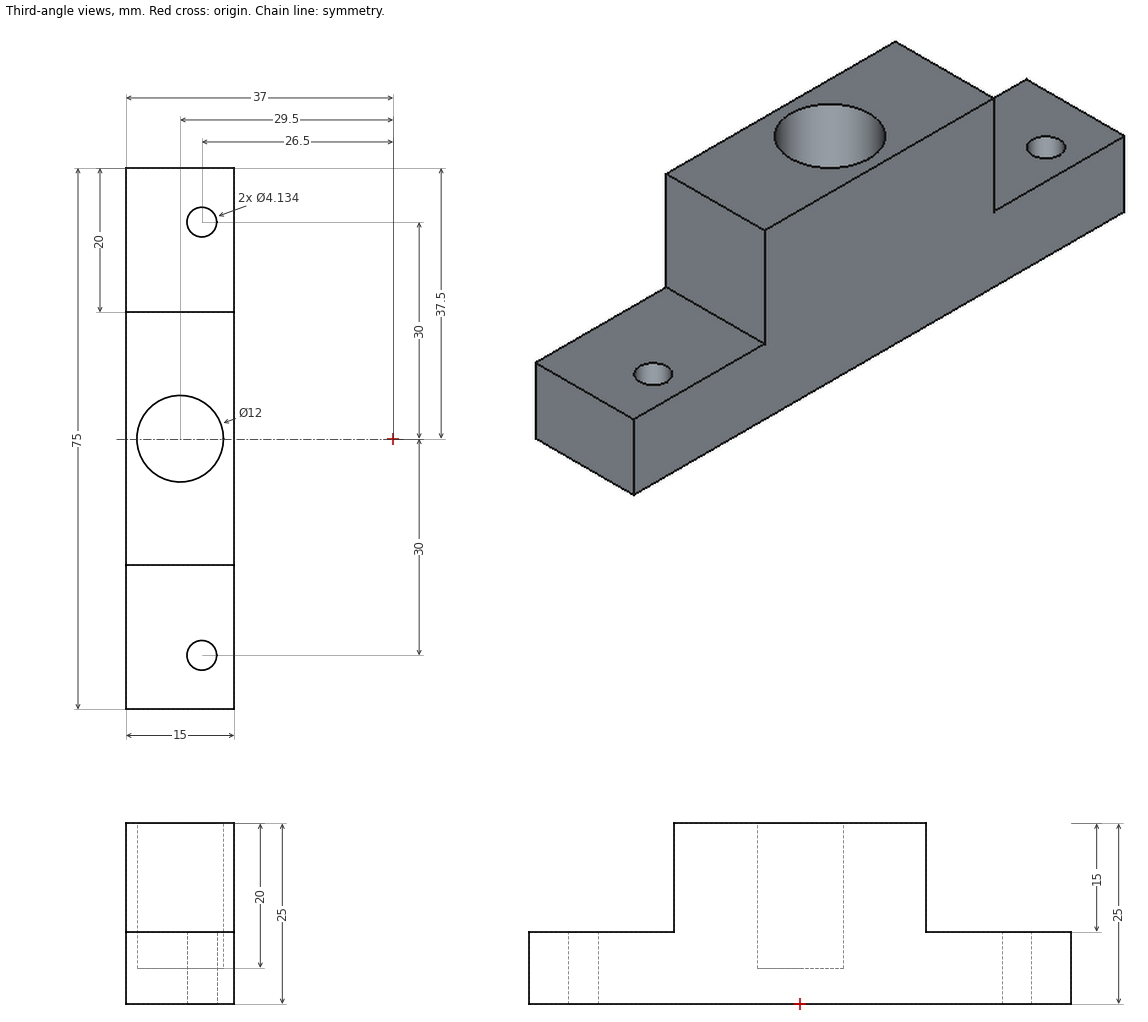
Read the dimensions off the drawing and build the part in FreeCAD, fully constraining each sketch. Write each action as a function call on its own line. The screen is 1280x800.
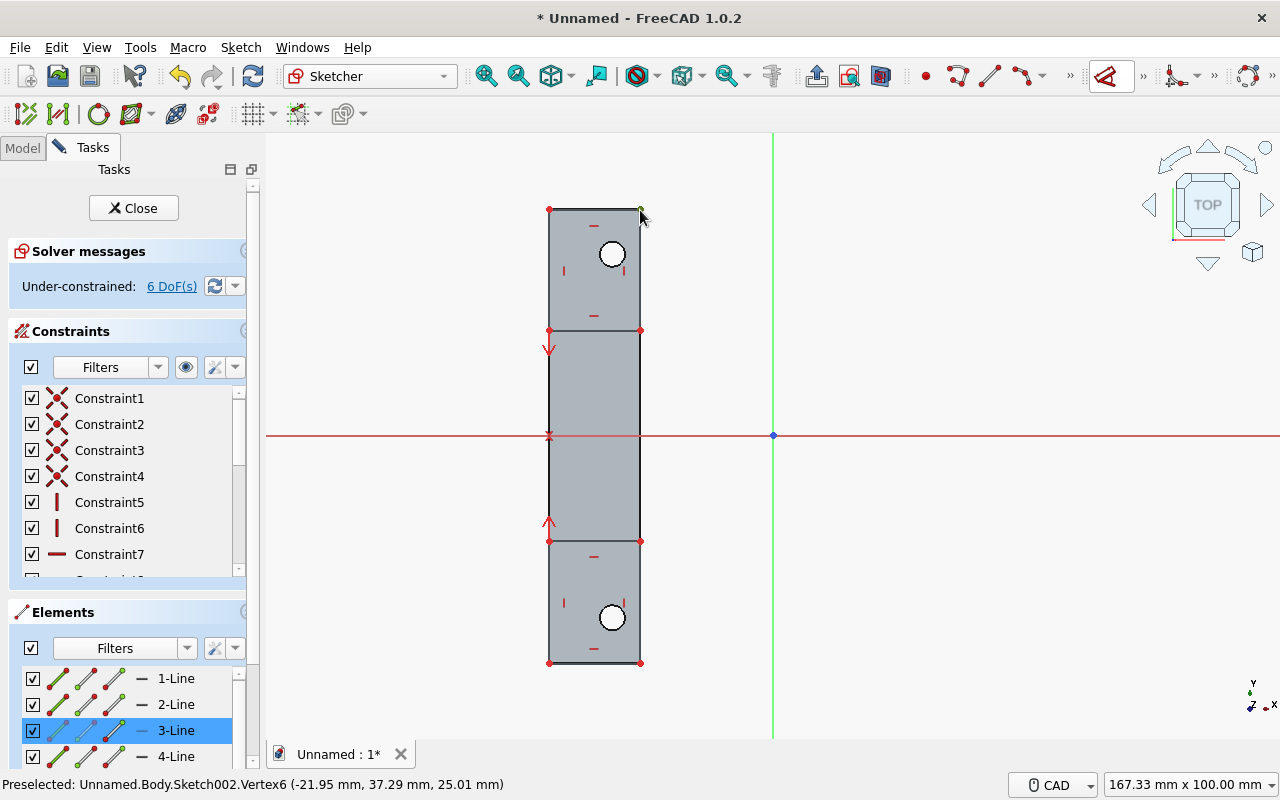
click(640, 664)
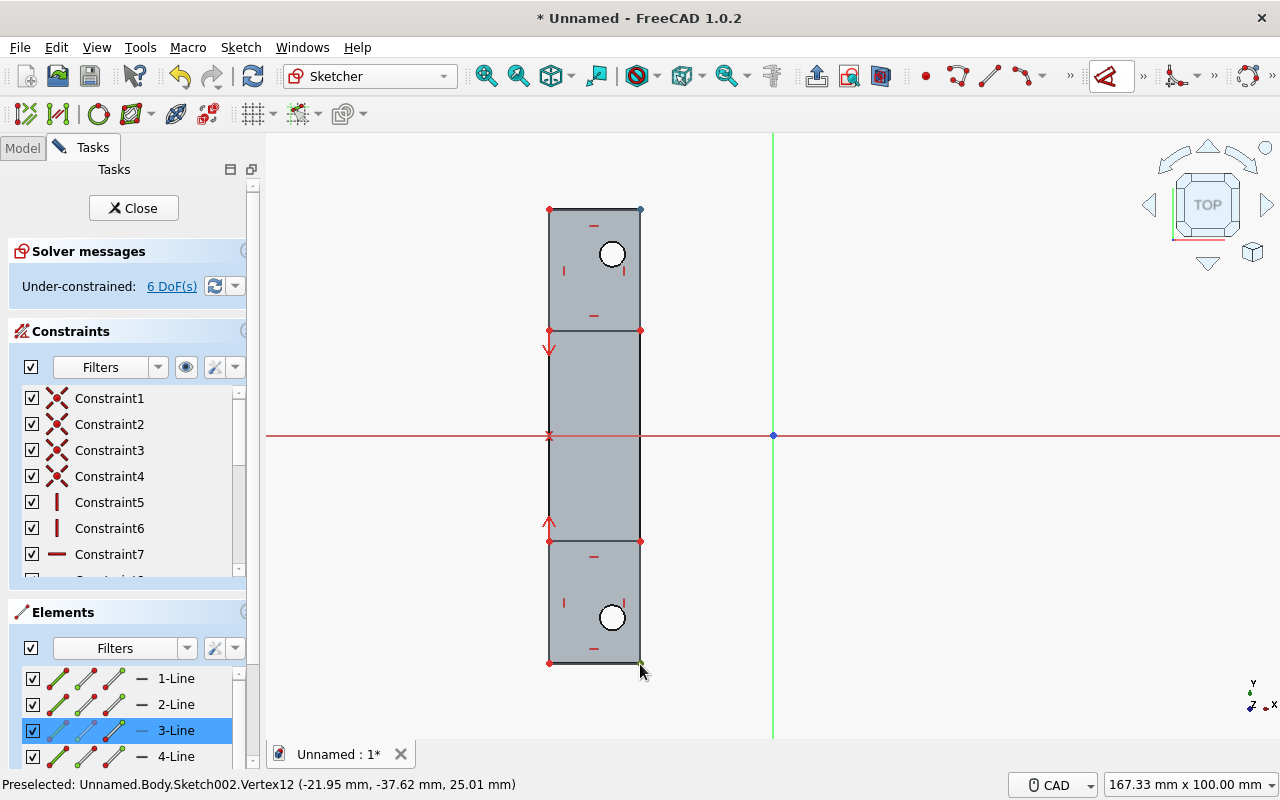
click(353, 436)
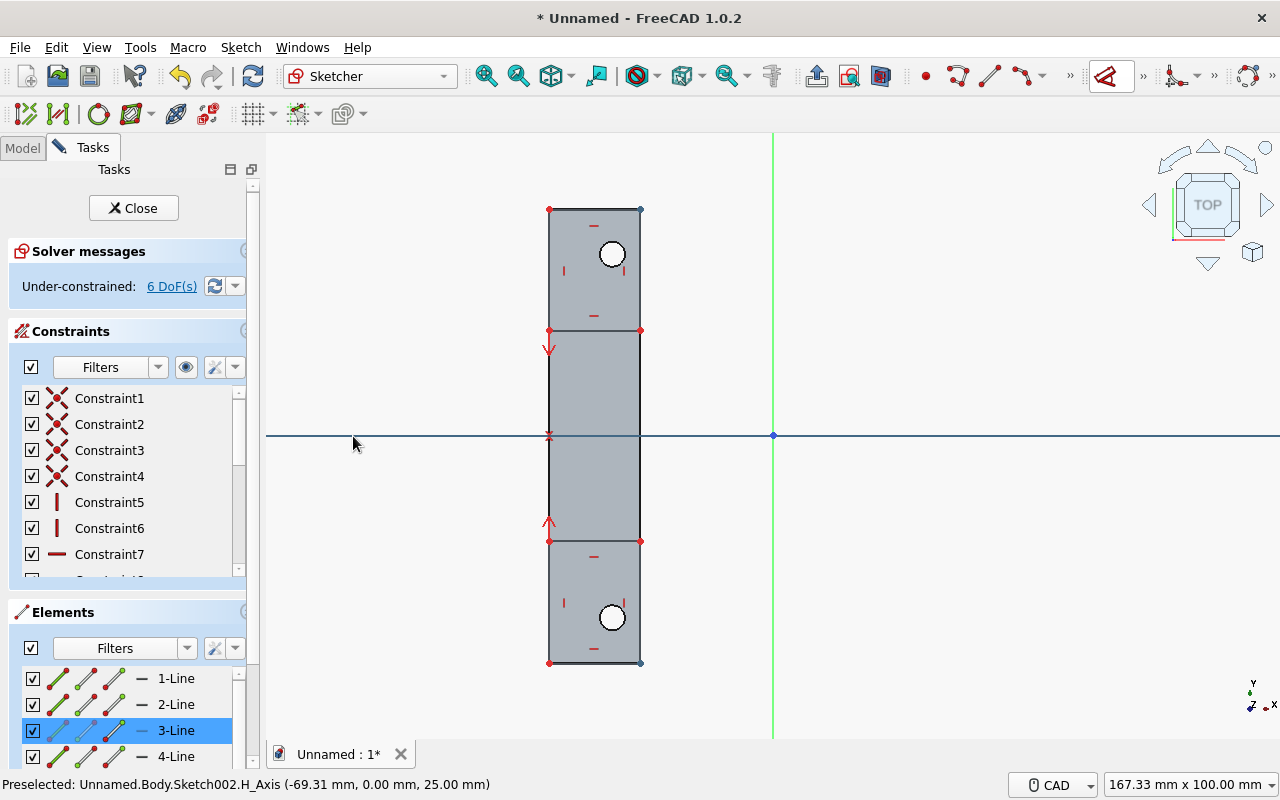
key(s)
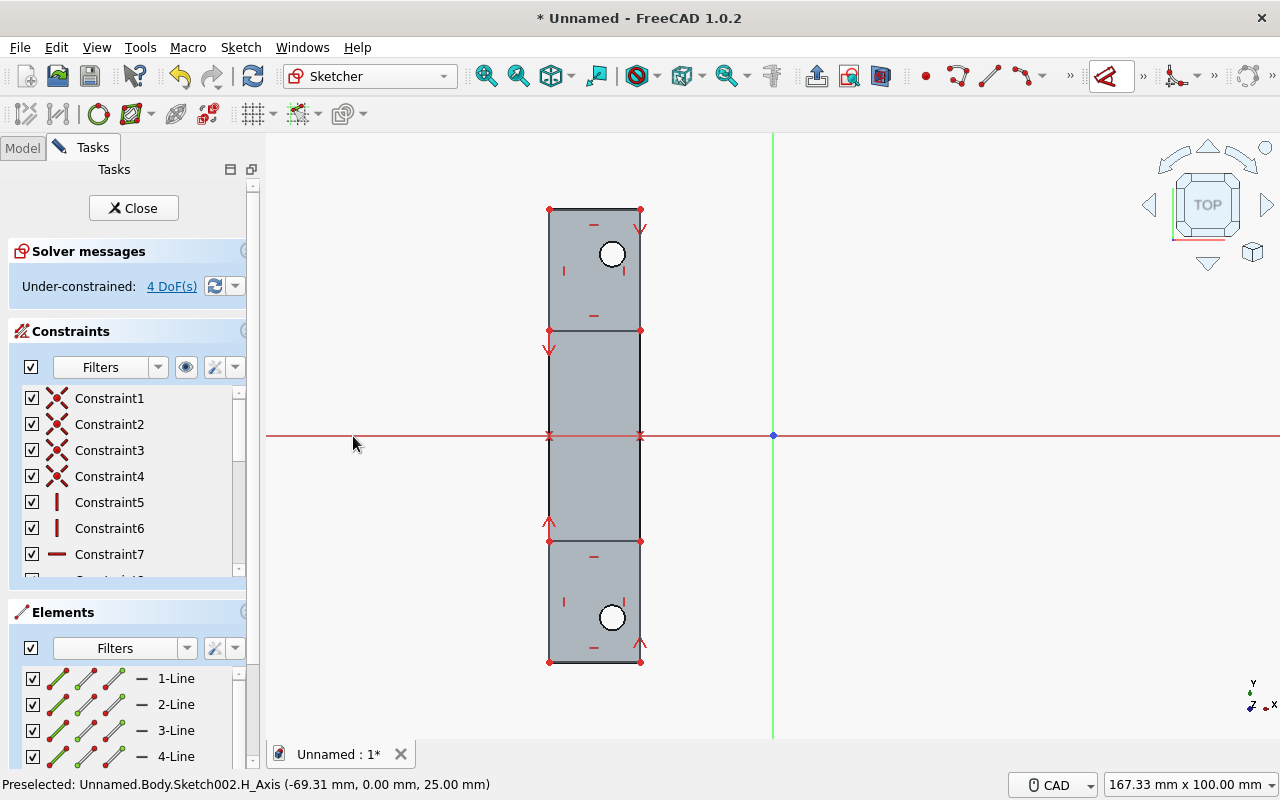
click(549, 246)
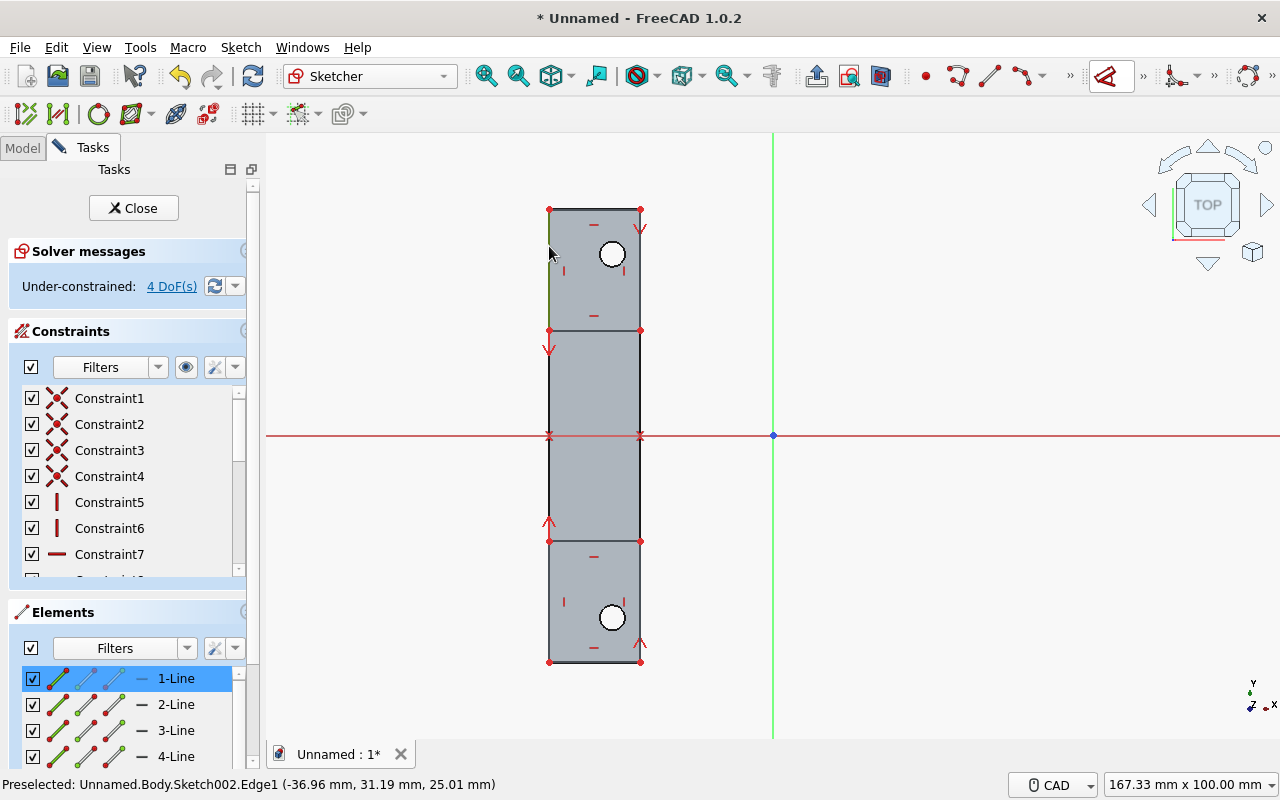
key(i)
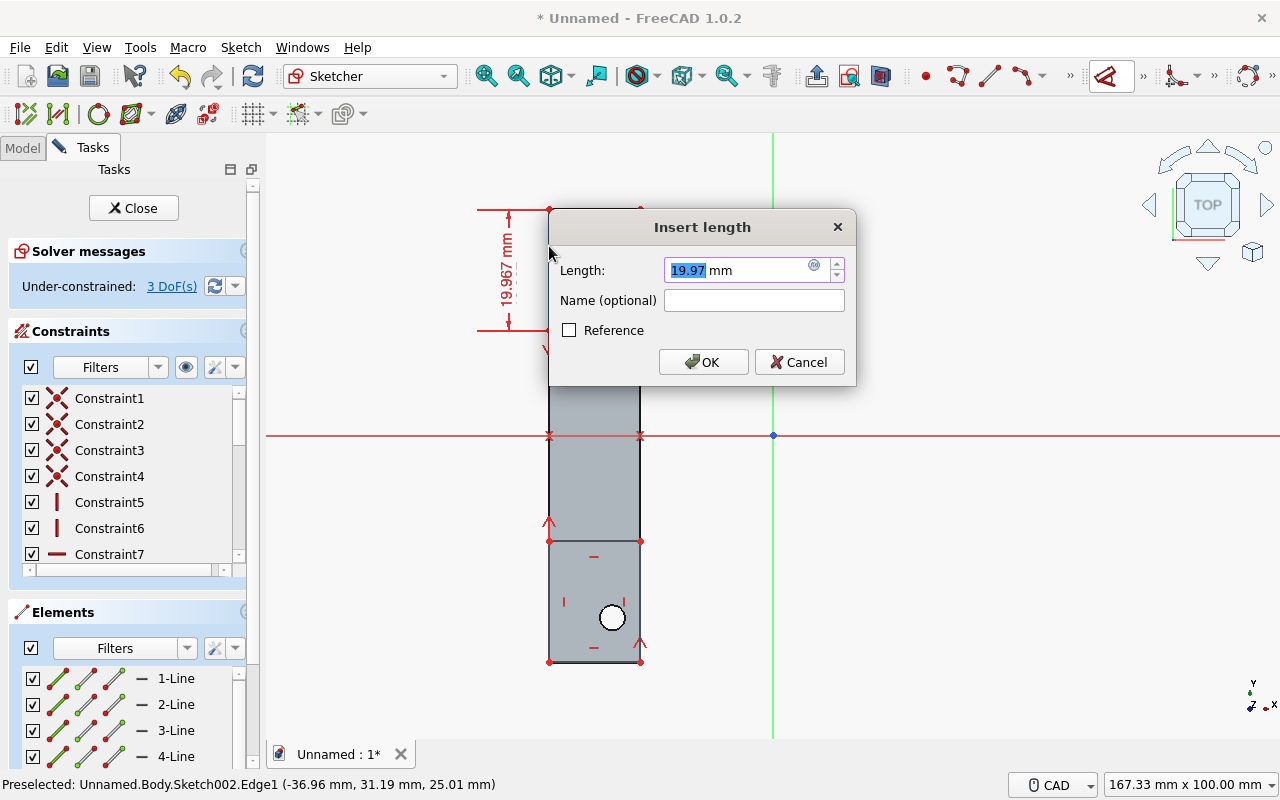
text(20)
key(Return)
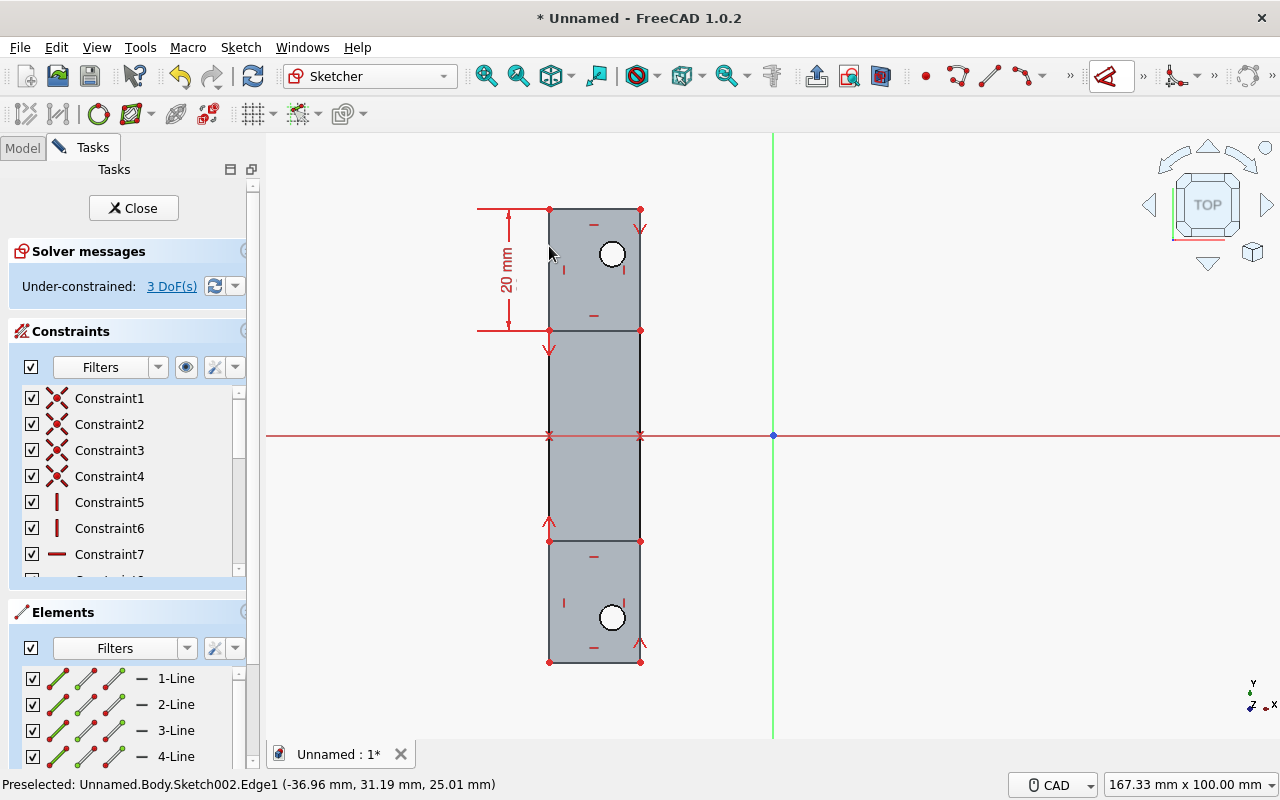
click(576, 331)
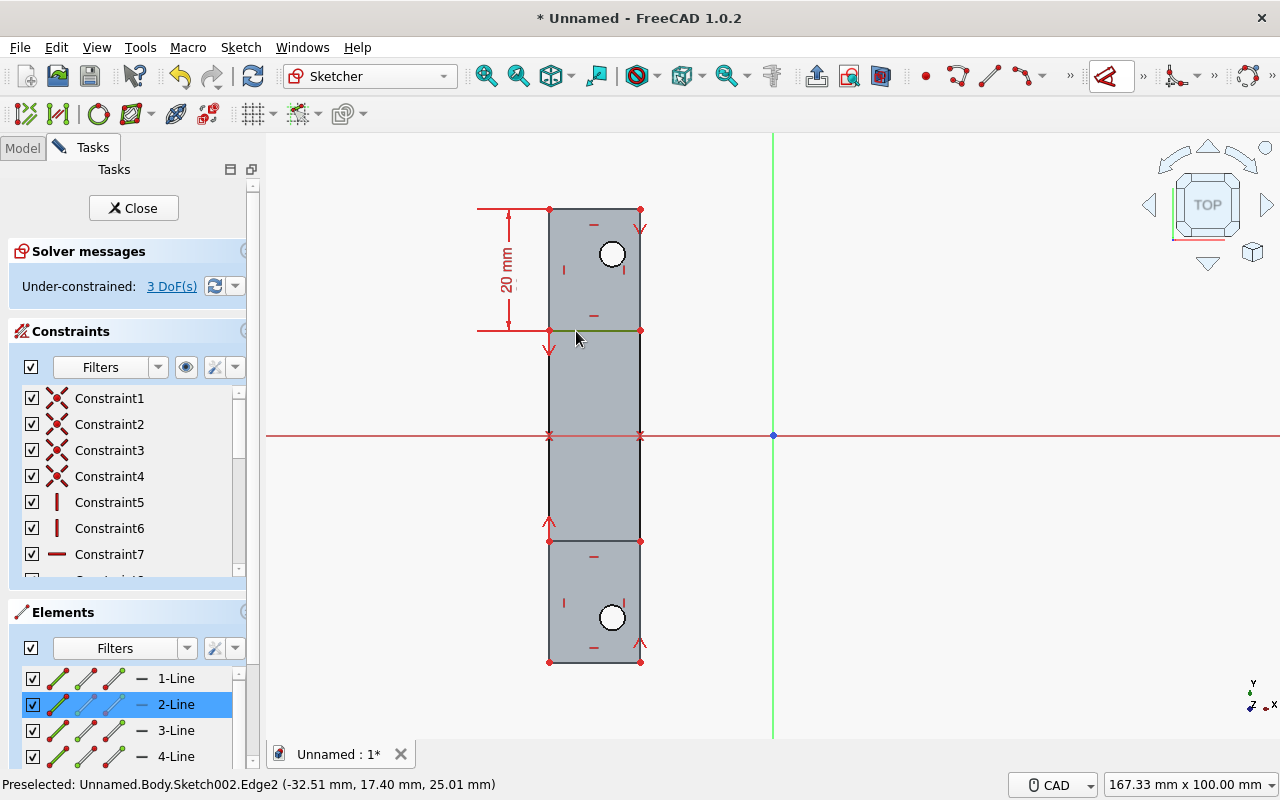
click(1128, 76)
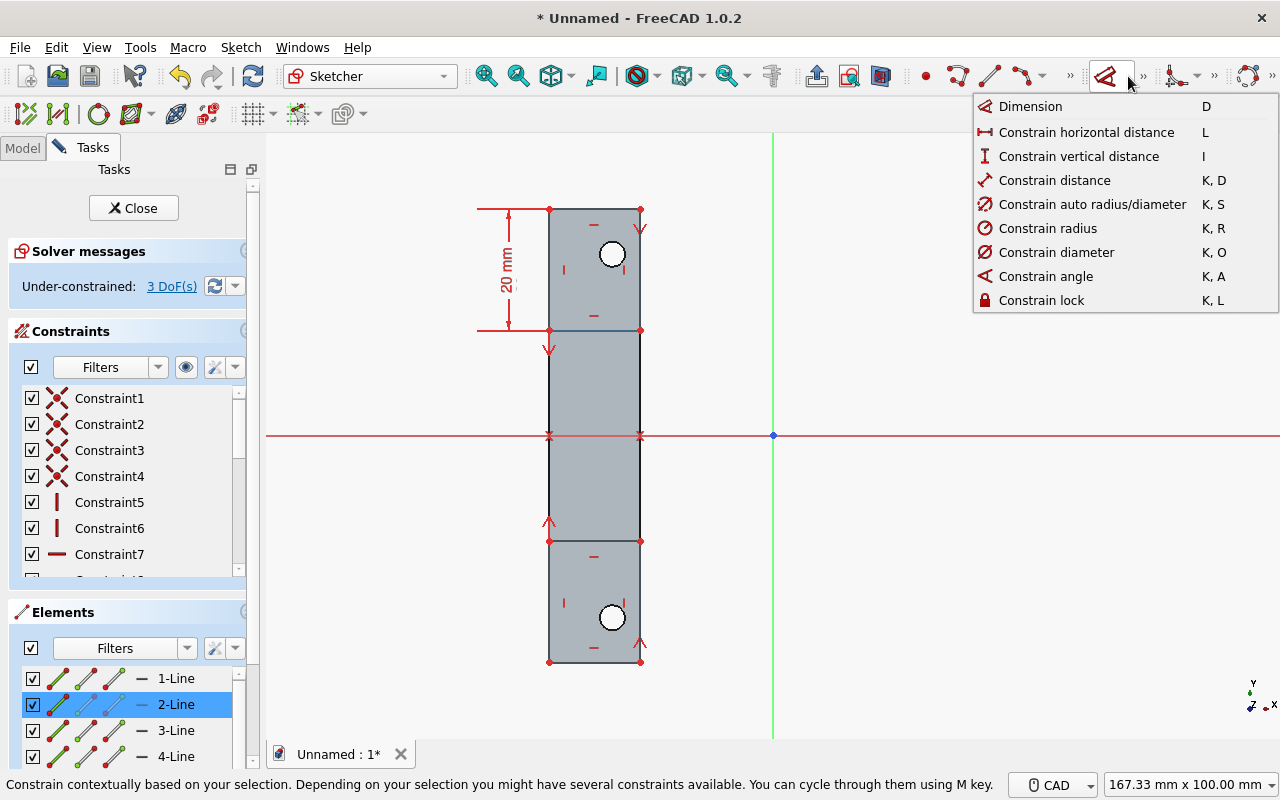
click(1126, 132)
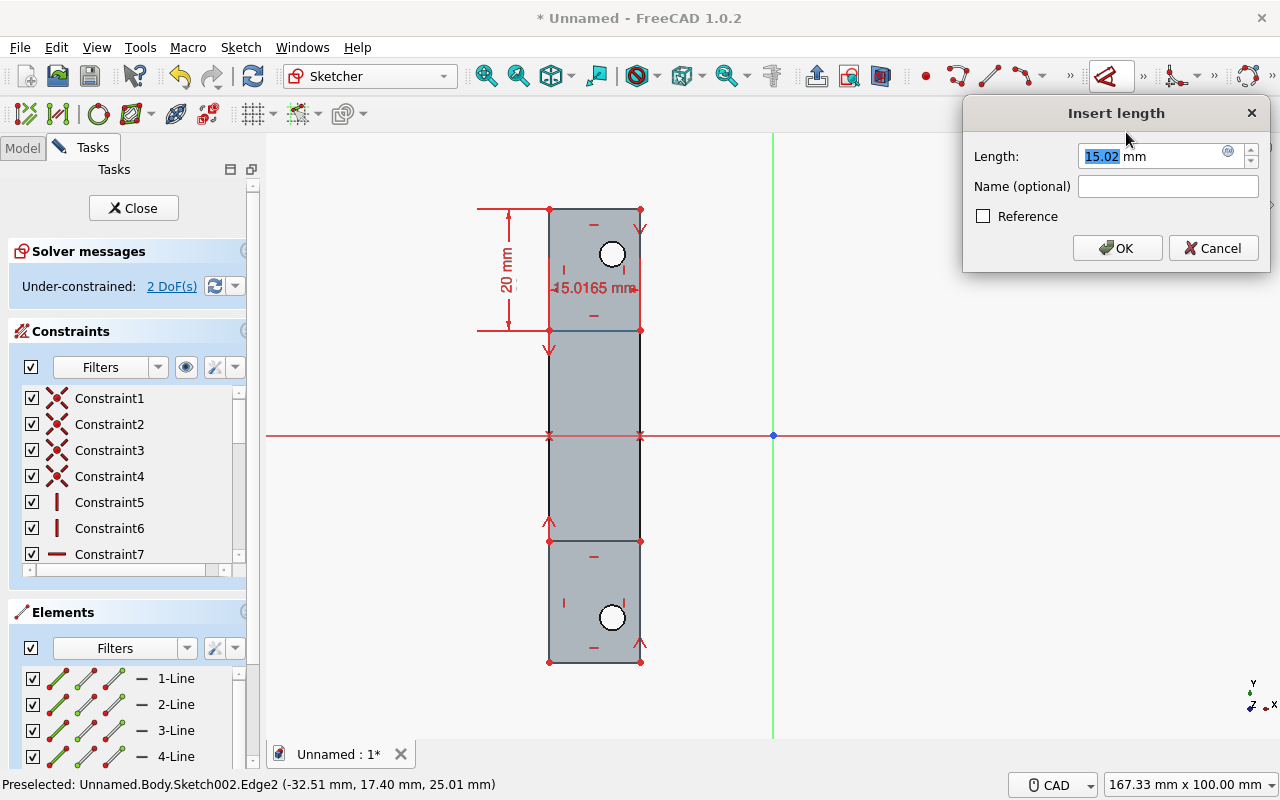
text(15)
key(Return)